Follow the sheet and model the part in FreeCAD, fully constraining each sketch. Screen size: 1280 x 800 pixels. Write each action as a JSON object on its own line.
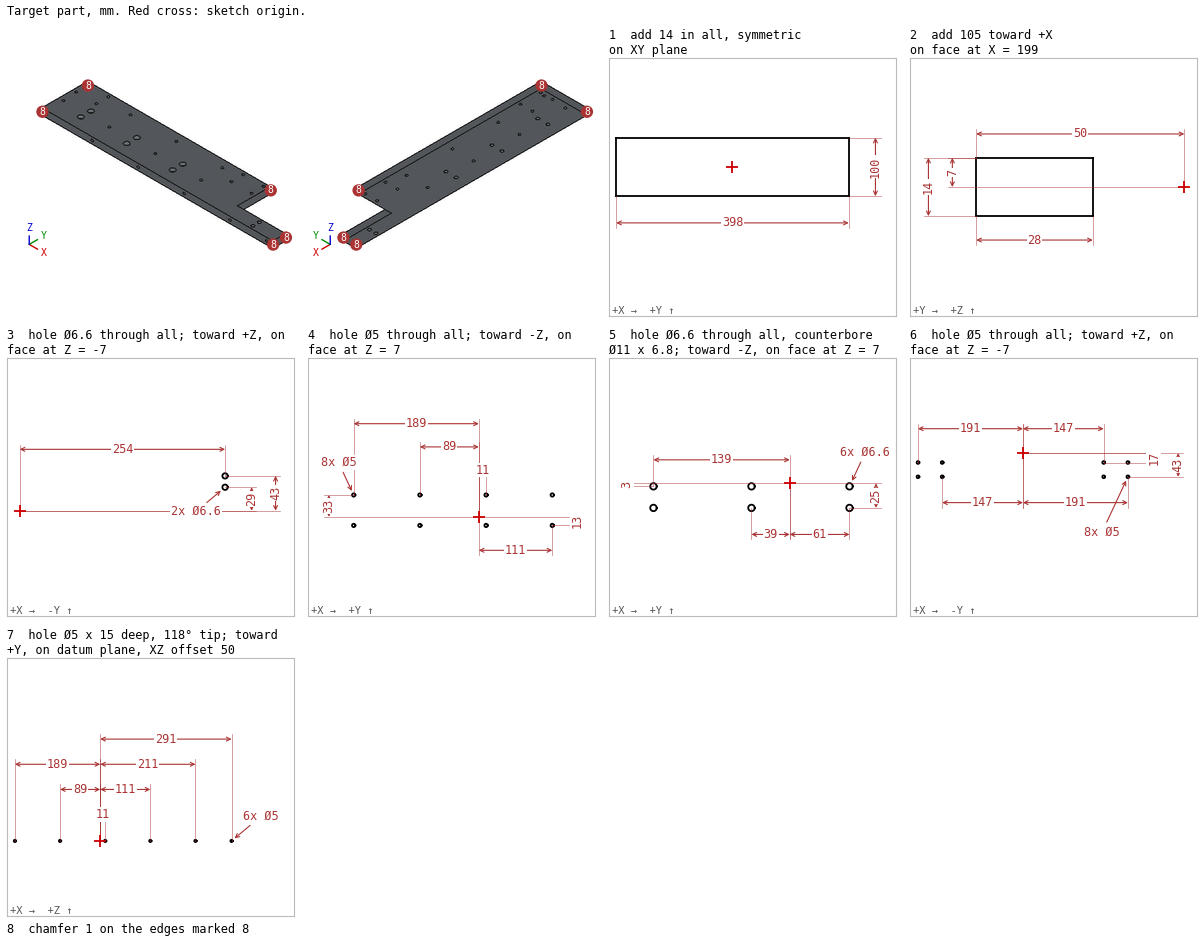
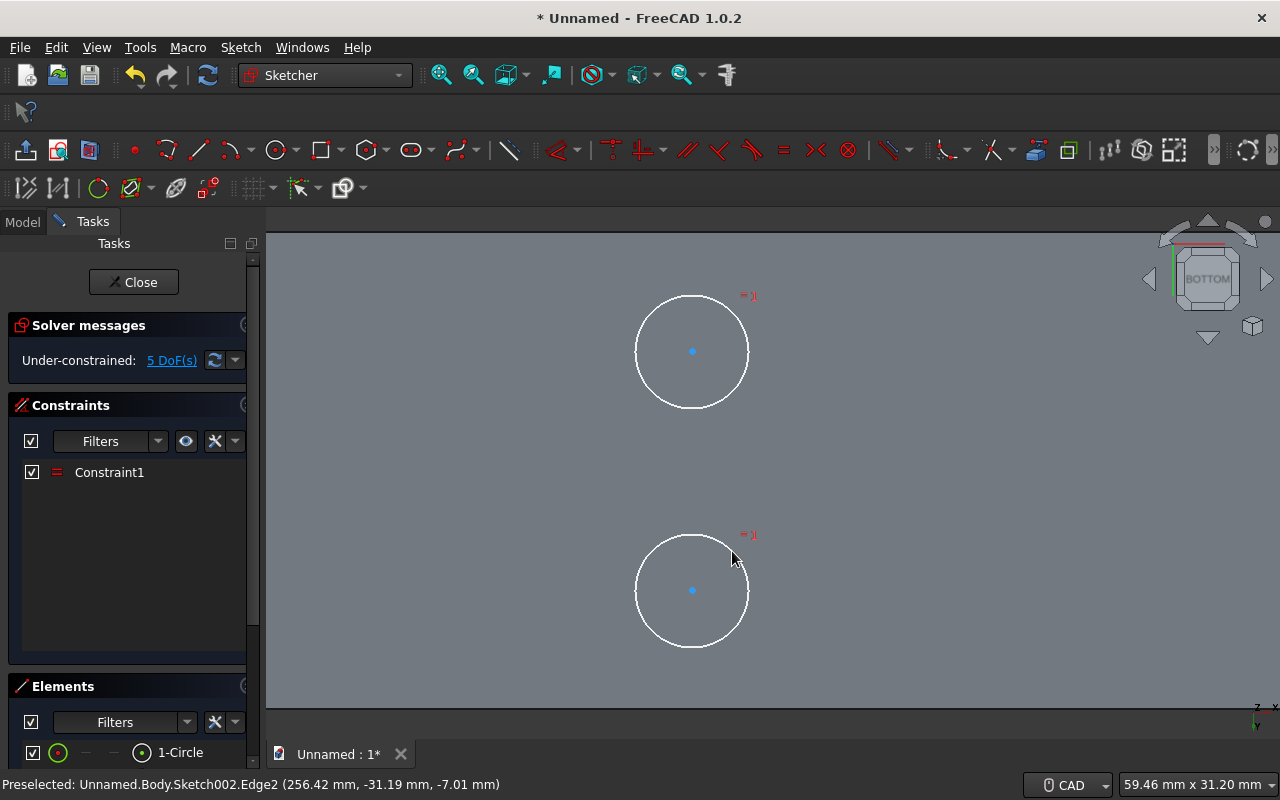
{"action": "left_click", "coordinate": [692, 352]}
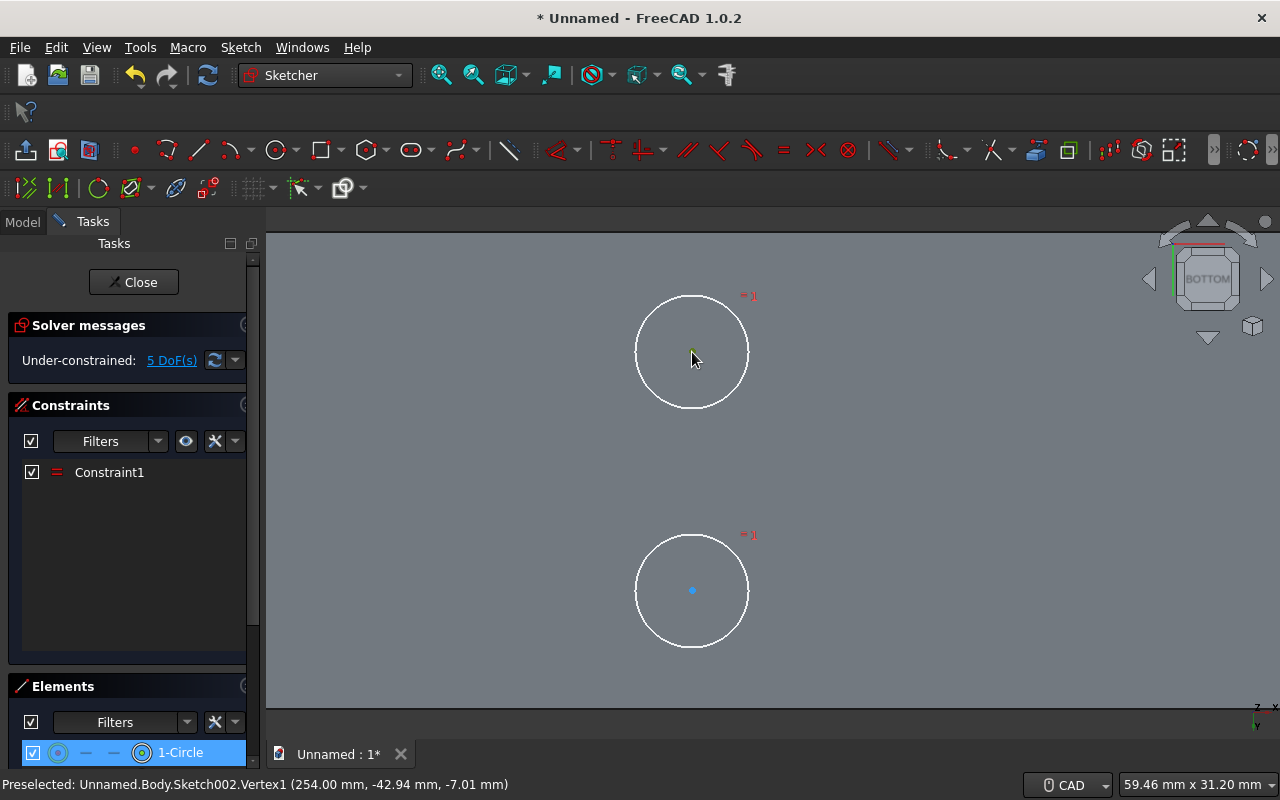
{"action": "left_click", "coordinate": [692, 591]}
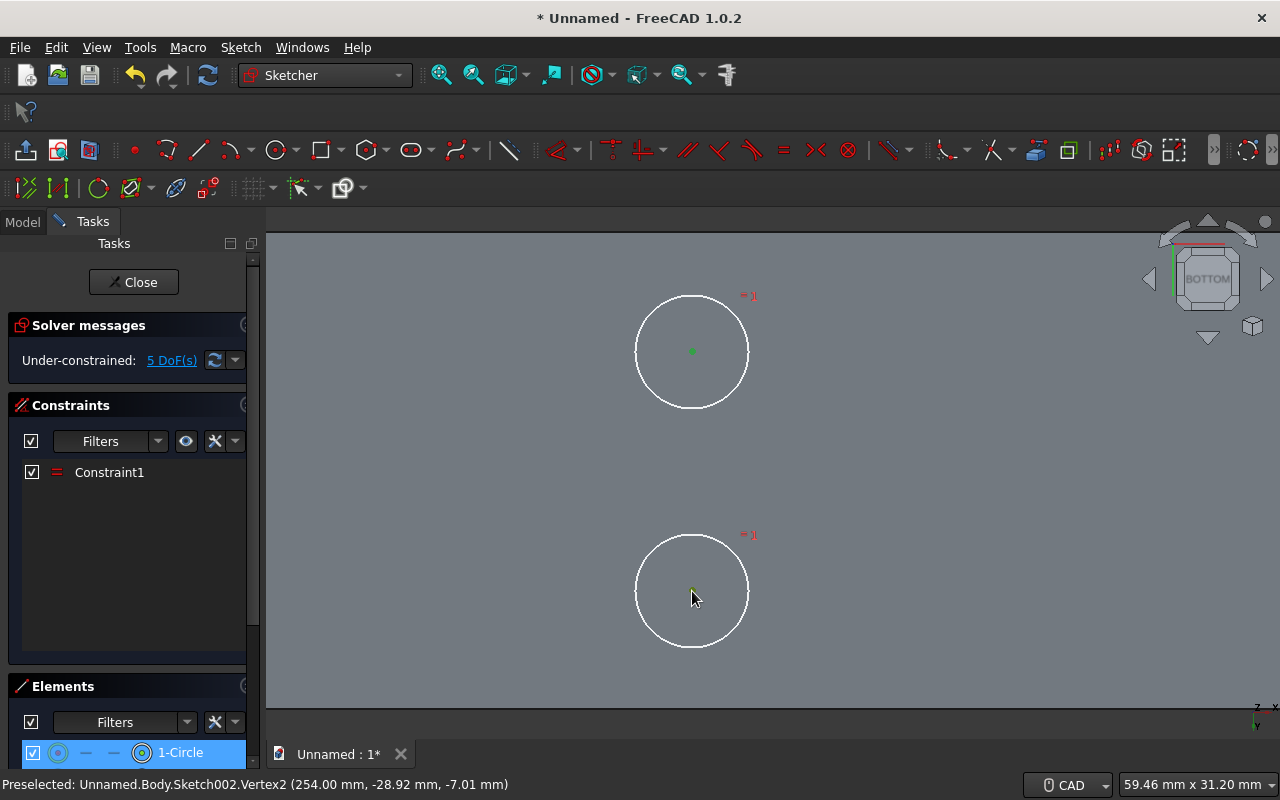
{"action": "left_click", "coordinate": [666, 150]}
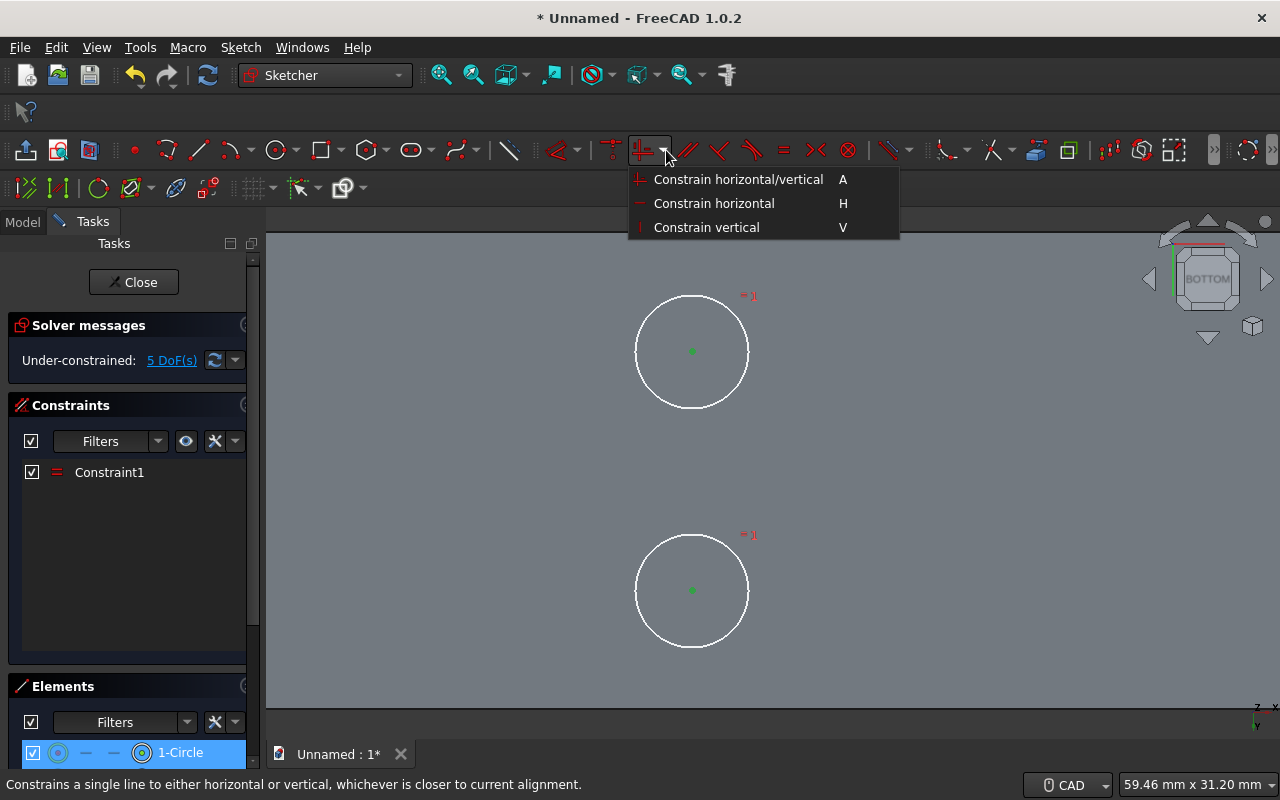
{"action": "left_click", "coordinate": [764, 227]}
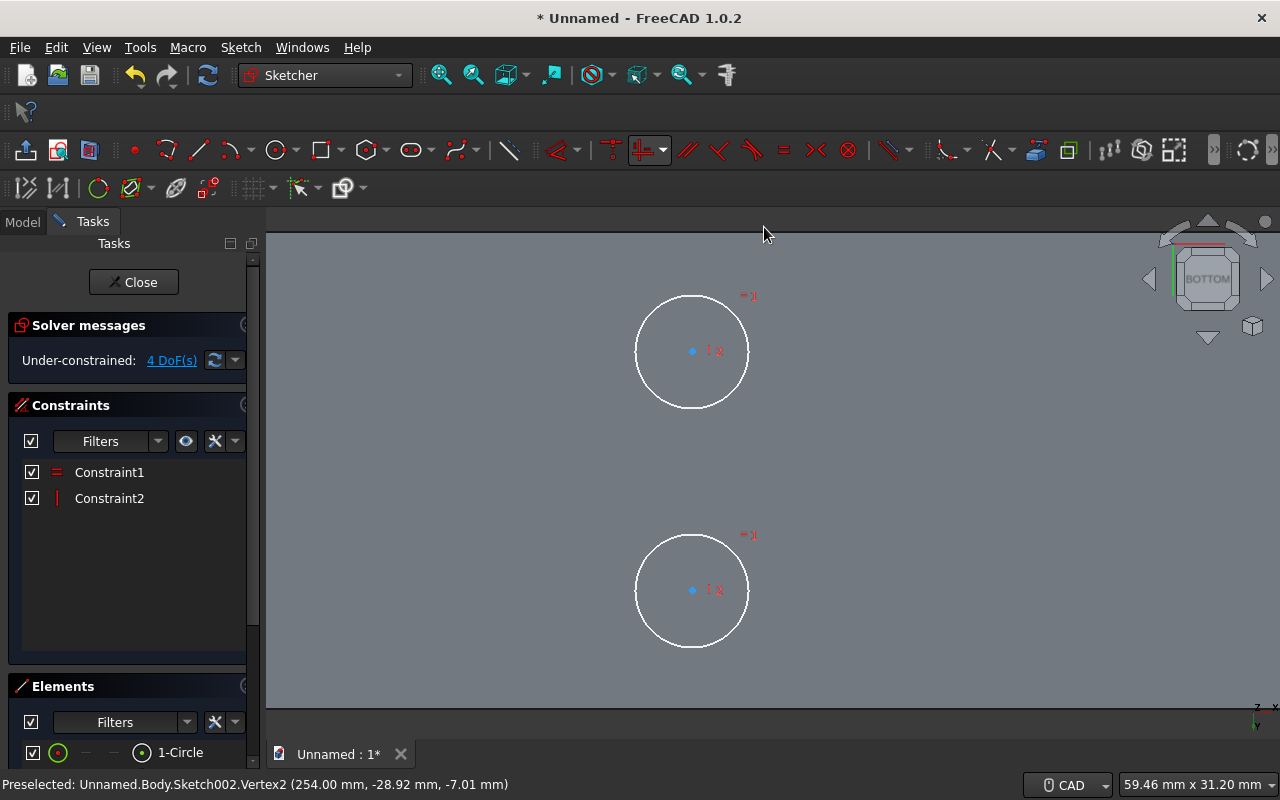
{"action": "left_click", "coordinate": [556, 150]}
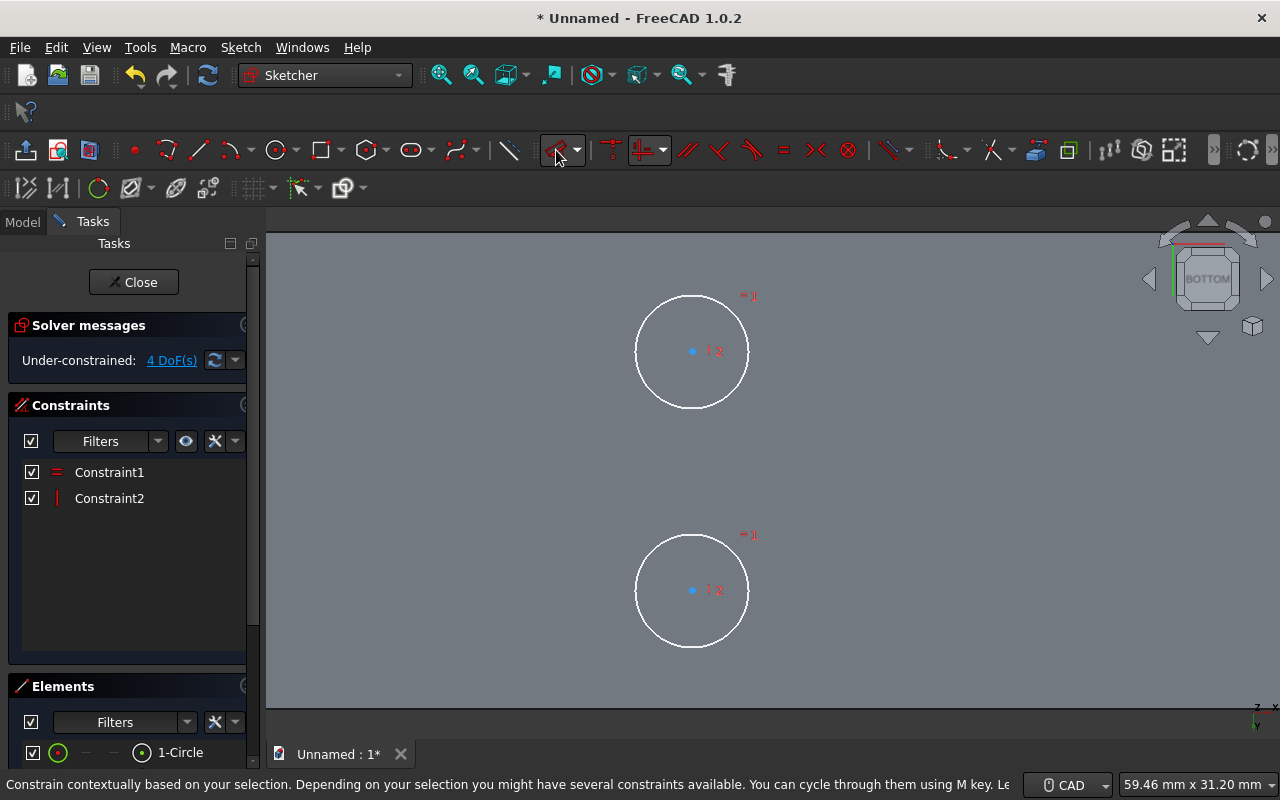
{"action": "left_click", "coordinate": [732, 312]}
{"action": "left_click", "coordinate": [755, 289]}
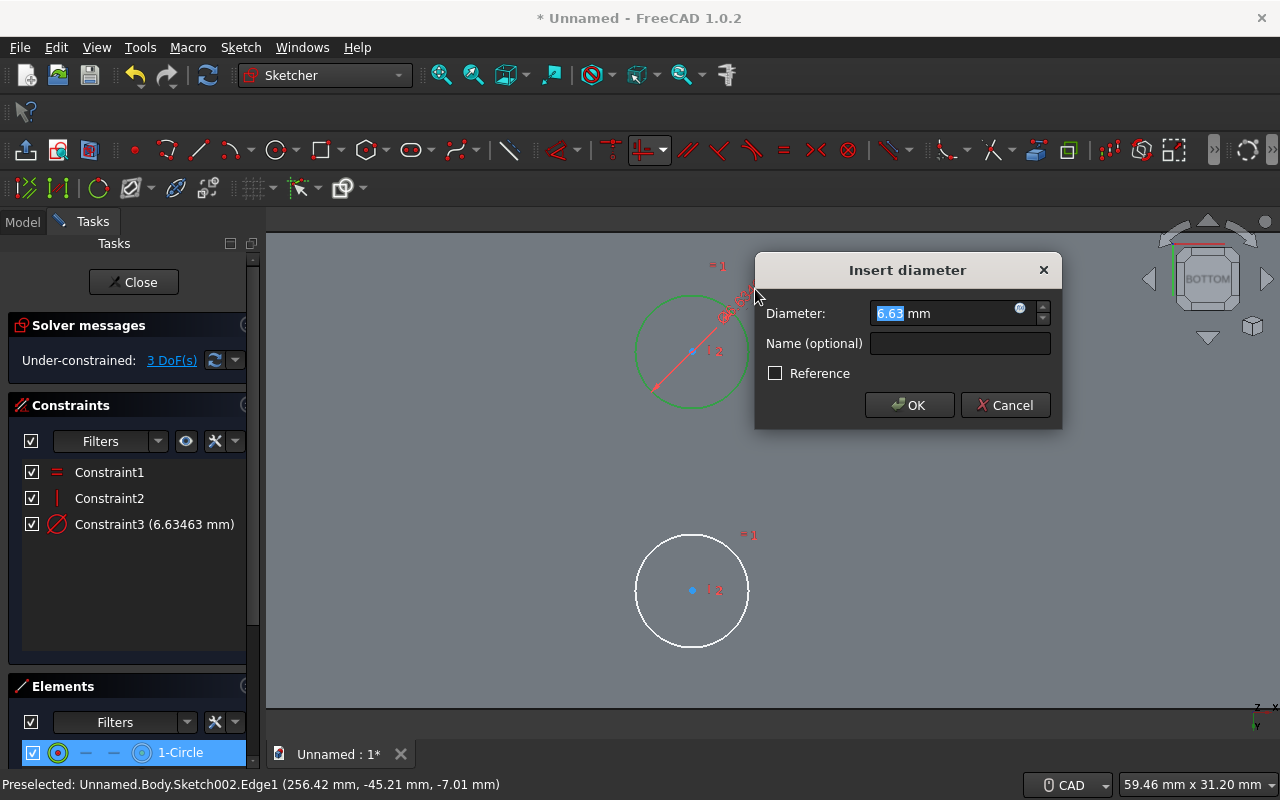
{"action": "type", "text": "6.6"}
{"action": "key", "text": "Return"}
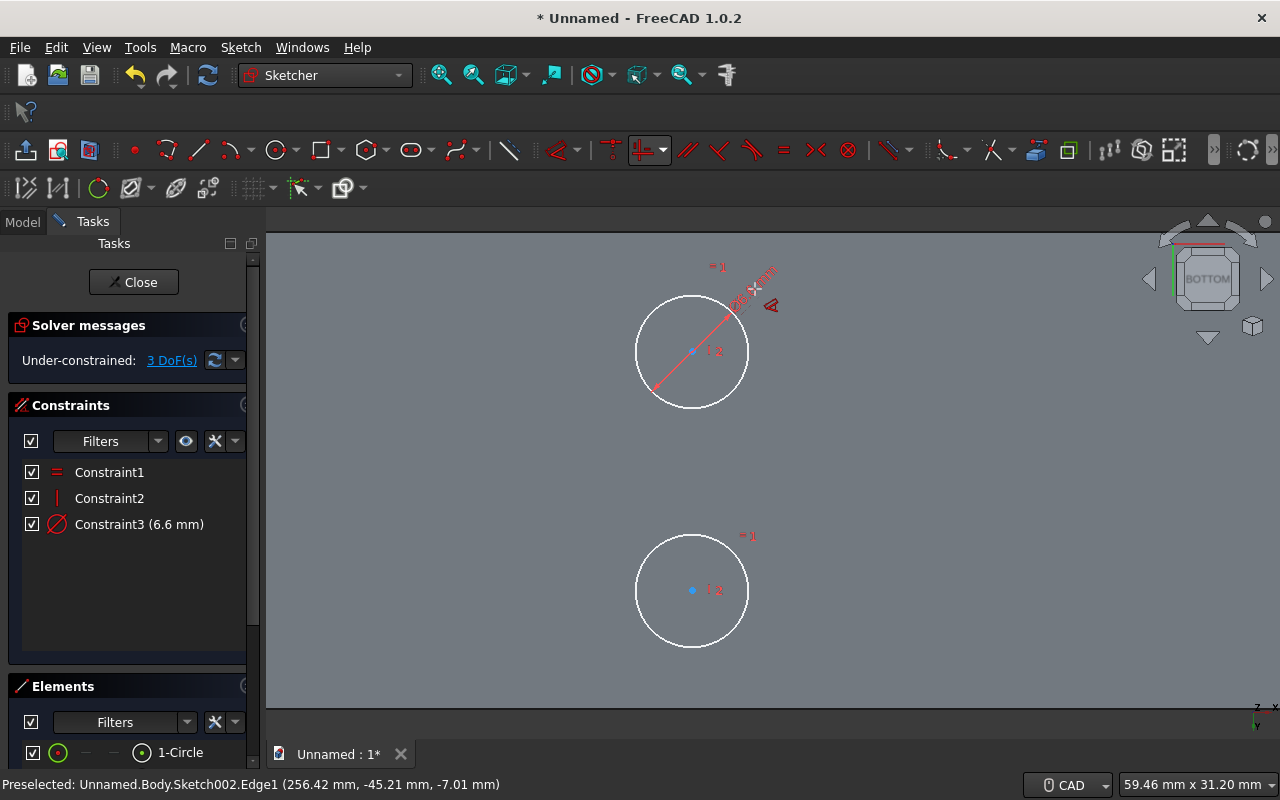
{"action": "left_click", "coordinate": [692, 352]}
{"action": "left_click", "coordinate": [726, 449]}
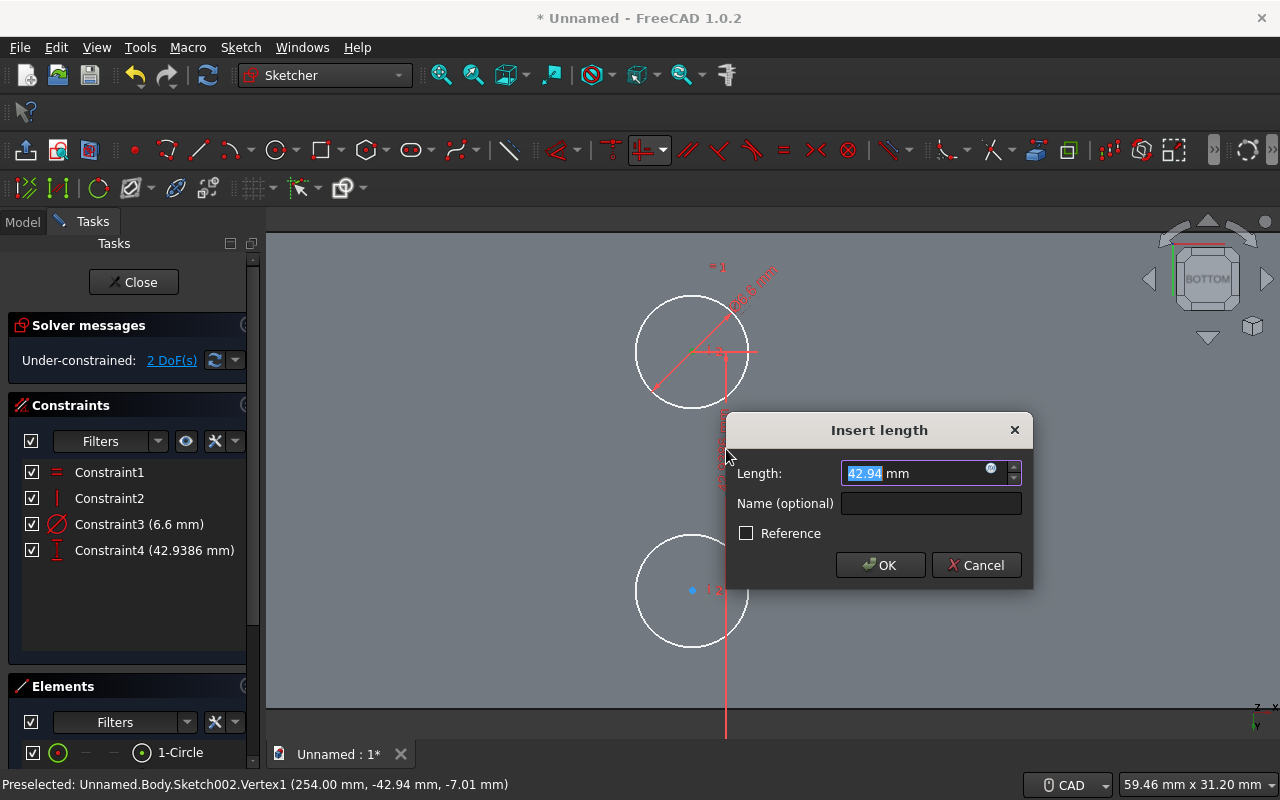
{"action": "type", "text": "43"}
{"action": "key", "text": "Return"}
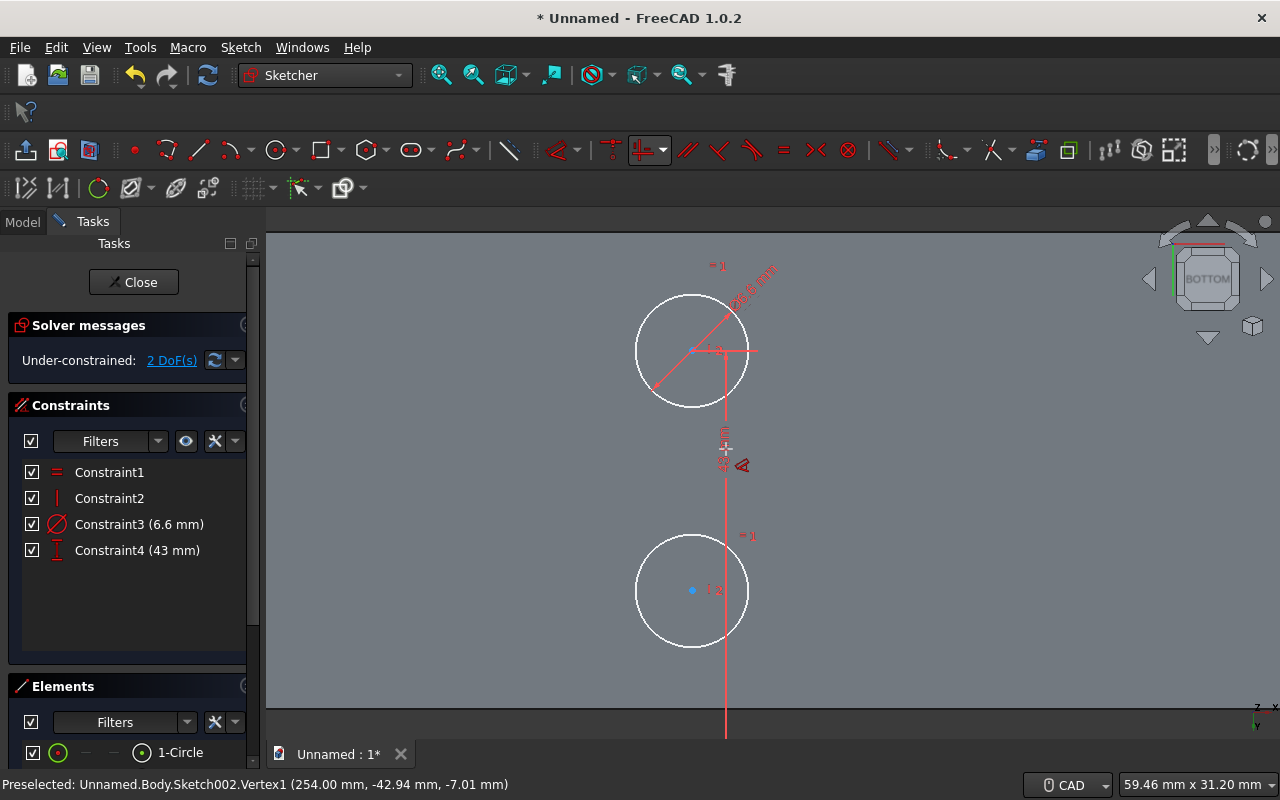
{"action": "left_click", "coordinate": [692, 591]}
{"action": "left_click", "coordinate": [726, 679]}